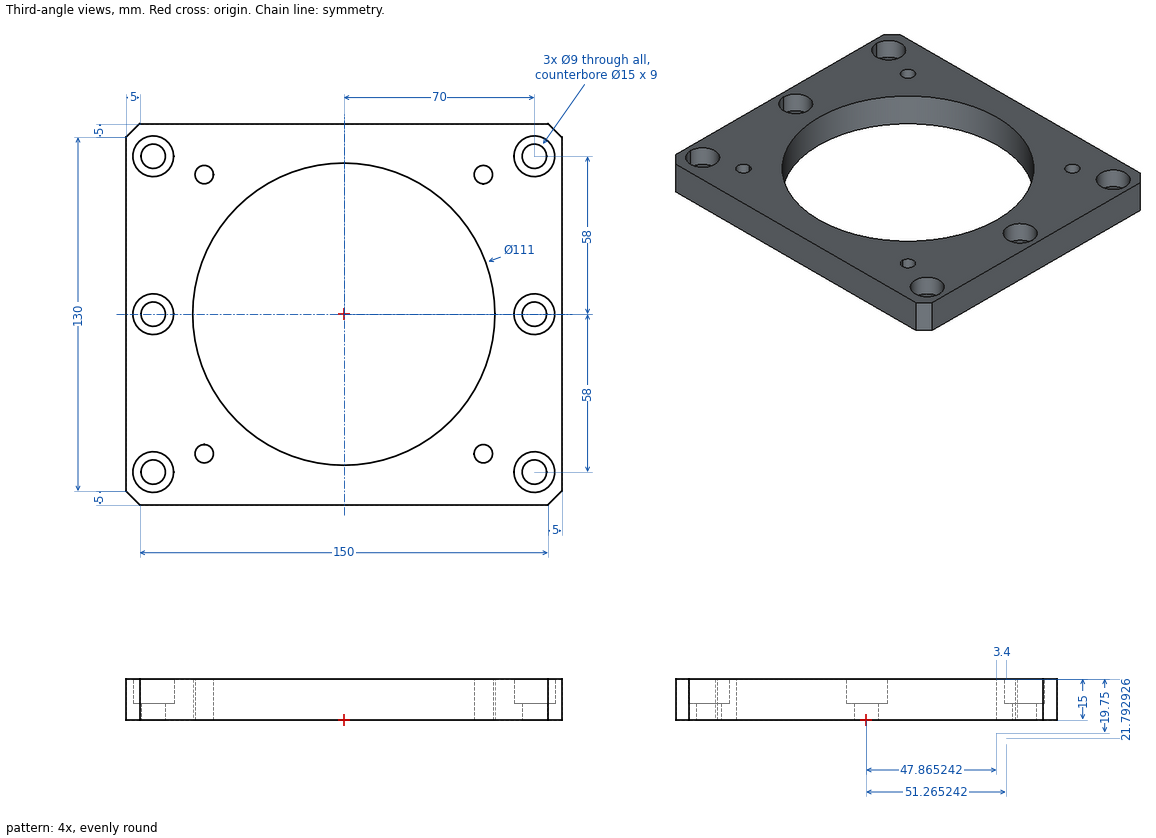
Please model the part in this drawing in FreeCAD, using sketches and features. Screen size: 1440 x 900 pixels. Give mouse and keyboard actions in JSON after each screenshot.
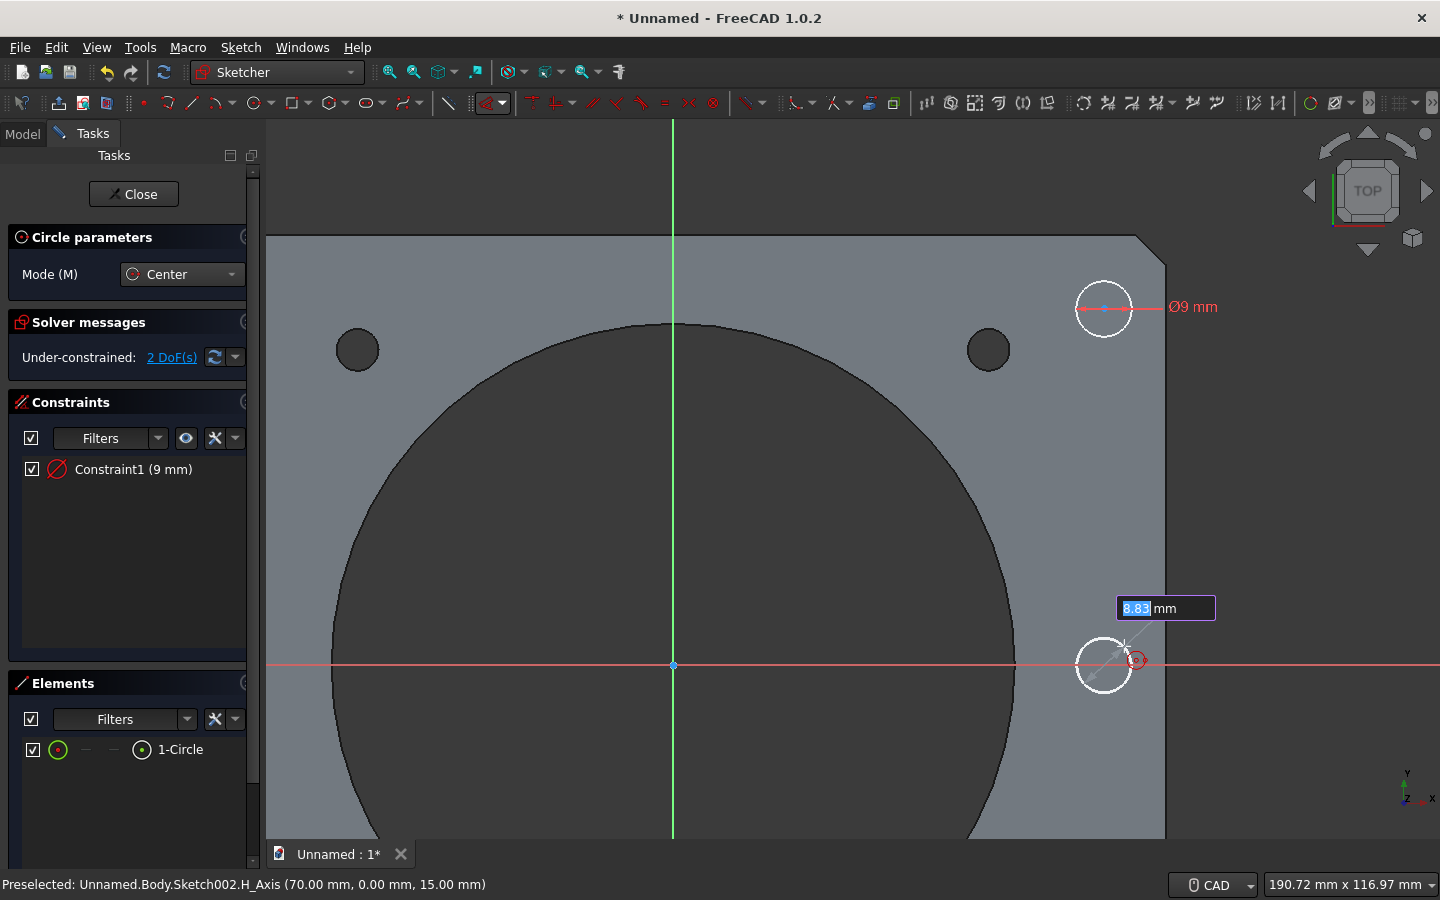
{"action": "type", "text": "9"}
{"action": "key", "text": "Return"}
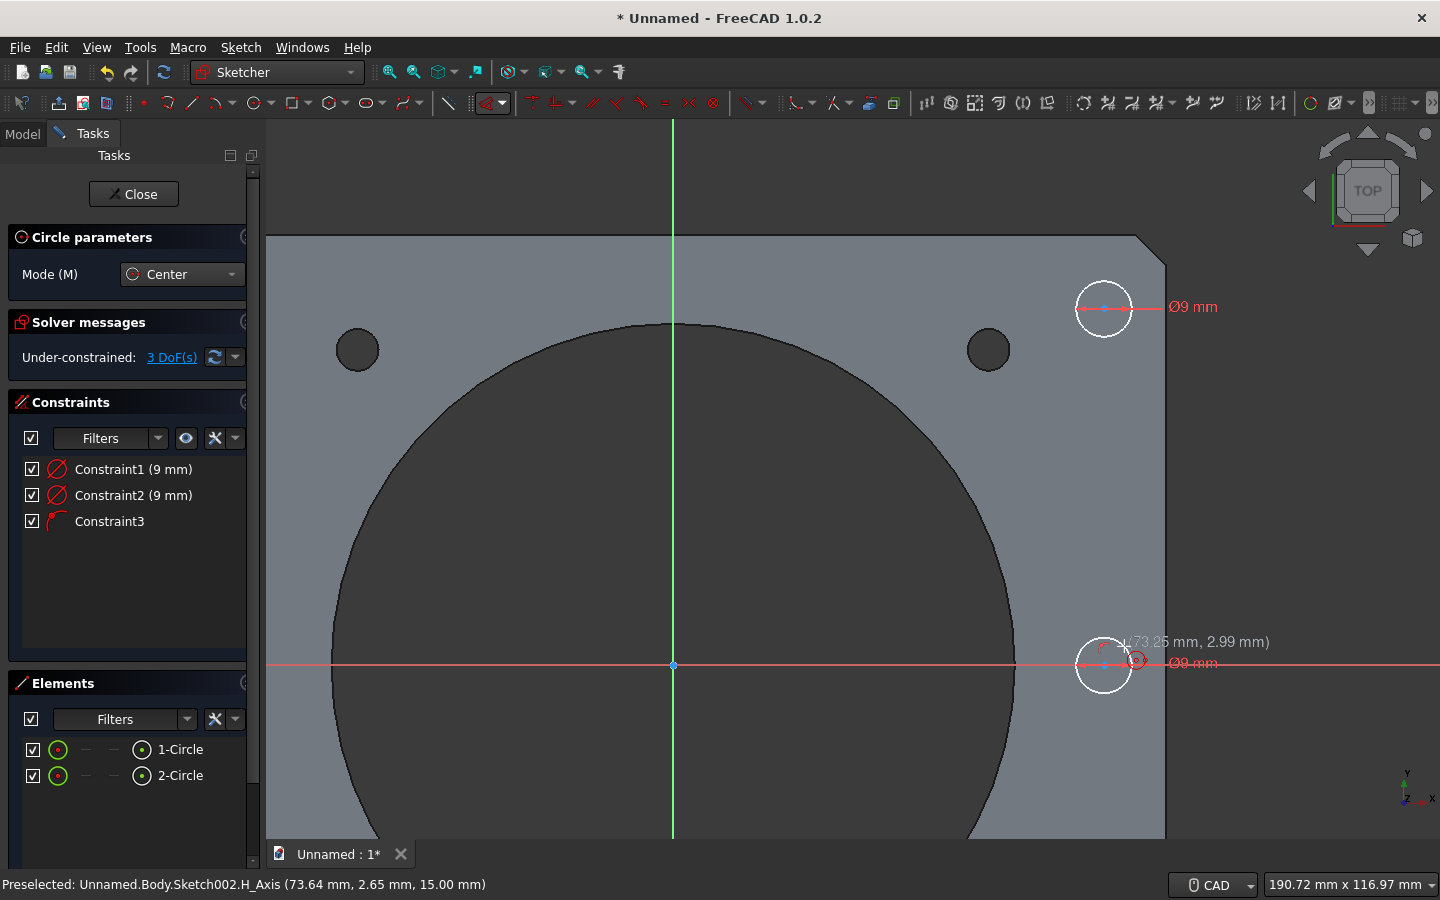
{"action": "scroll", "coordinate": [545, 147], "scroll_direction": "down", "scroll_amount": 2}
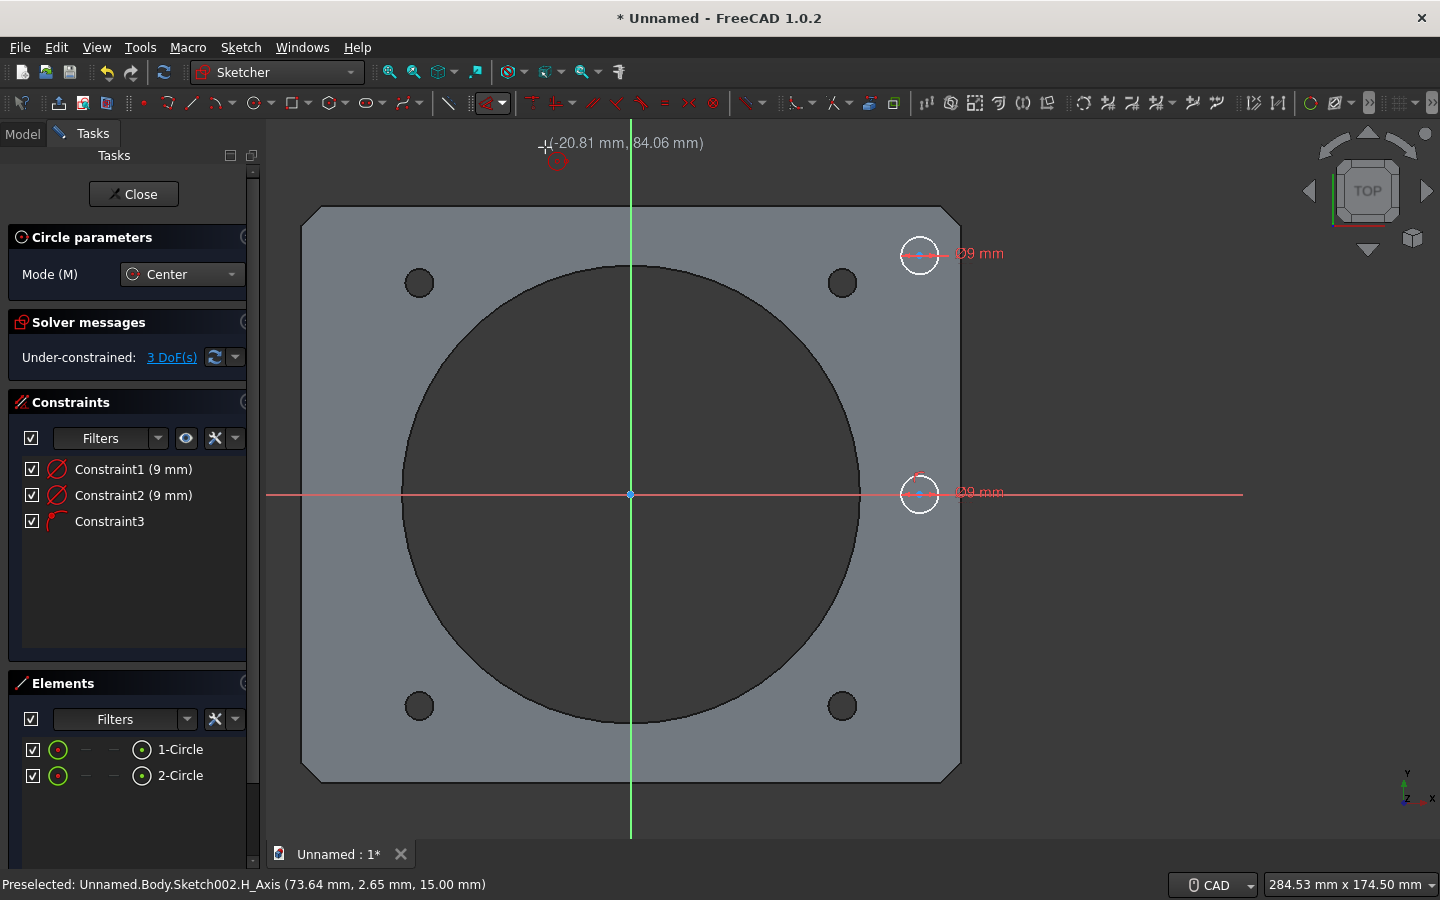
{"action": "scroll", "coordinate": [920, 734], "scroll_direction": "up", "scroll_amount": 2}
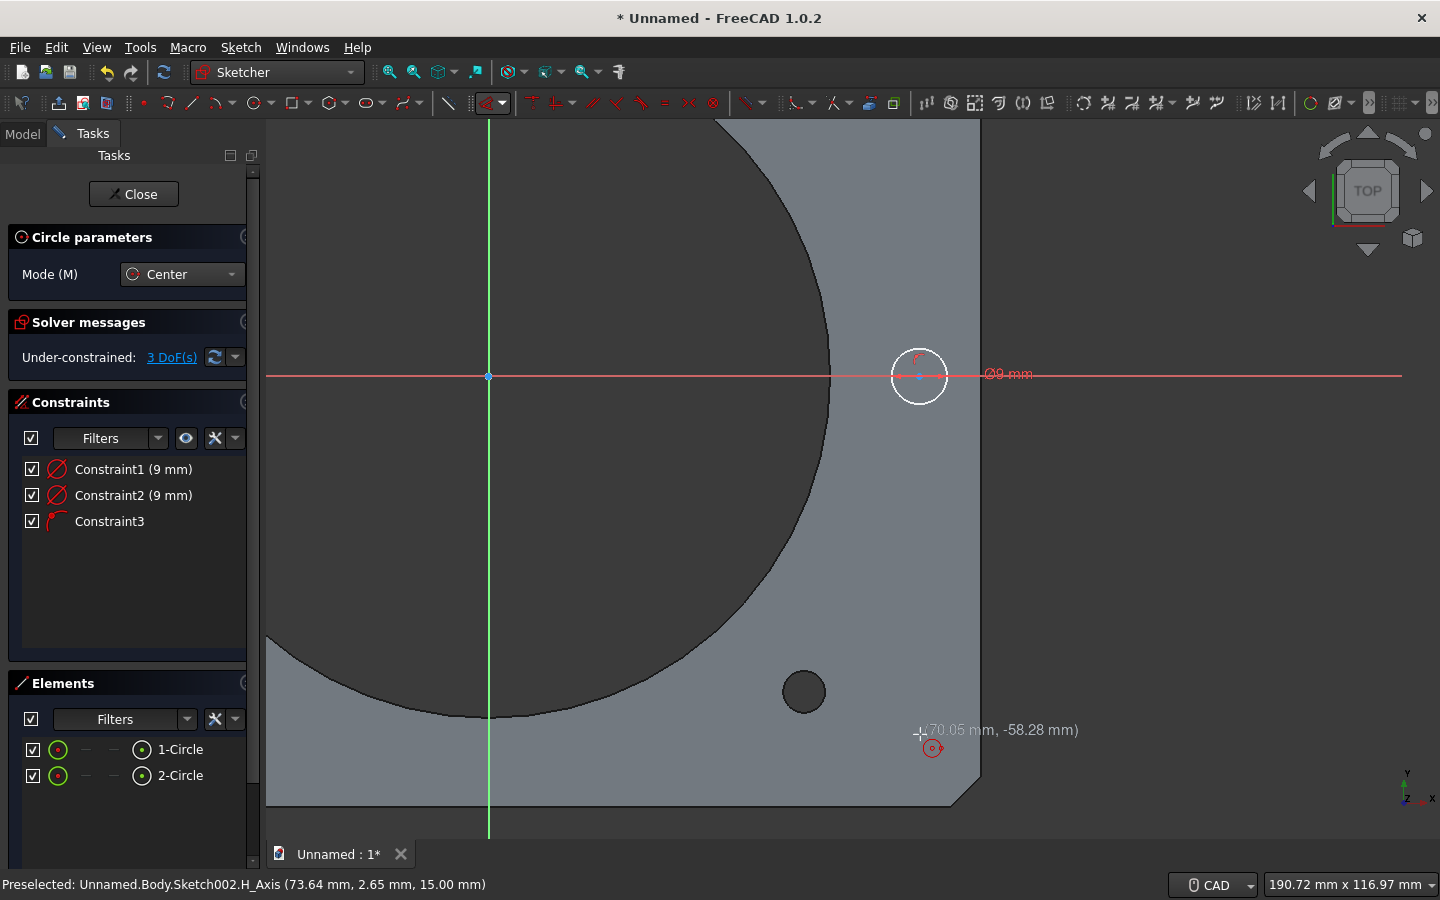
{"action": "left_click", "coordinate": [919, 733]}
{"action": "mouse_move", "coordinate": [939, 714]}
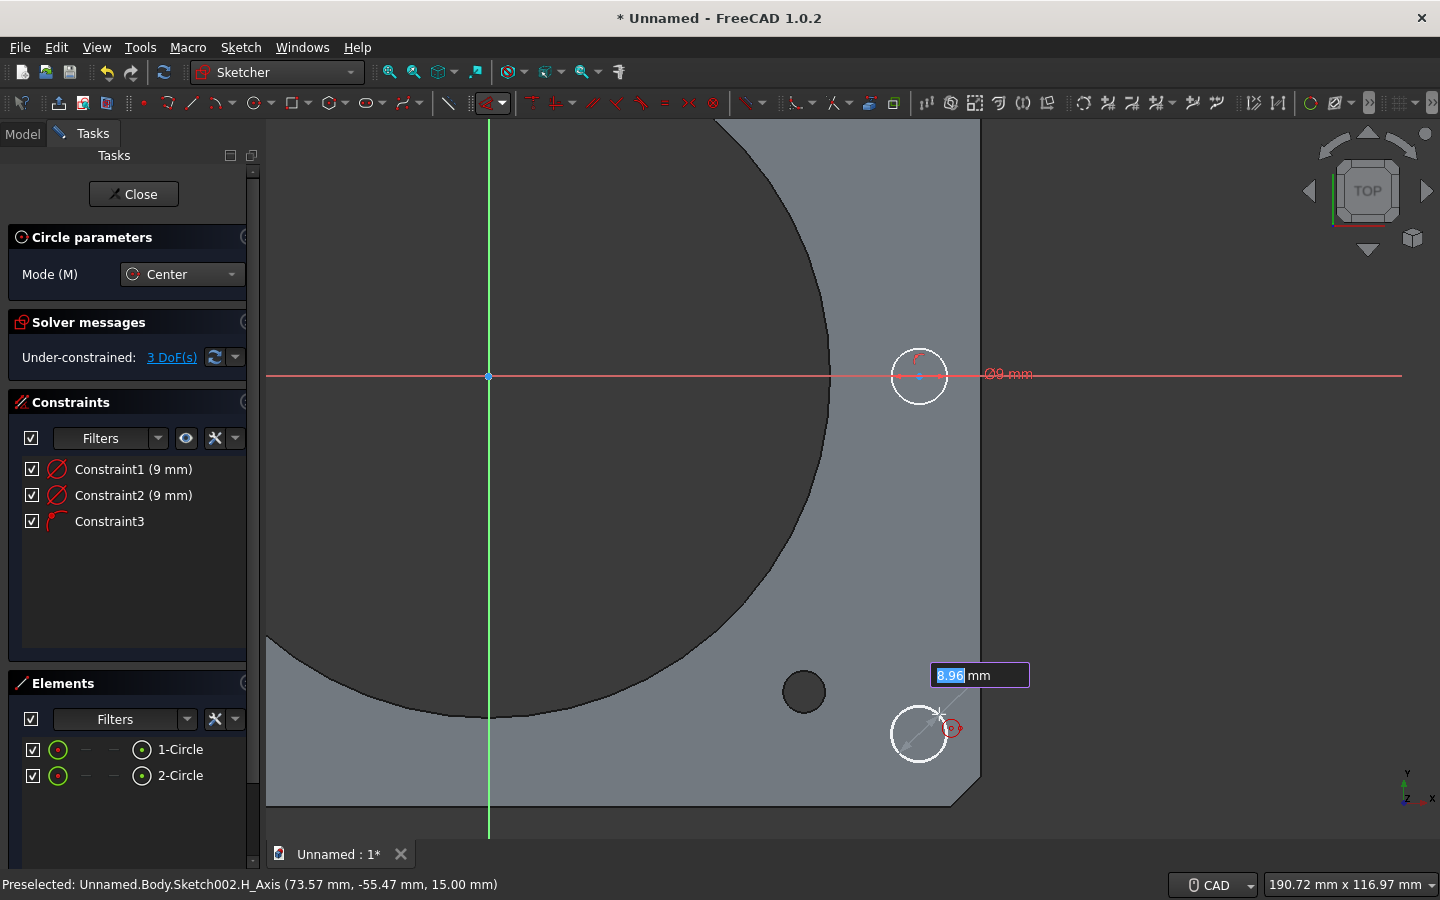
{"action": "type", "text": "9"}
{"action": "key", "text": "Return"}
{"action": "key", "text": "Escape"}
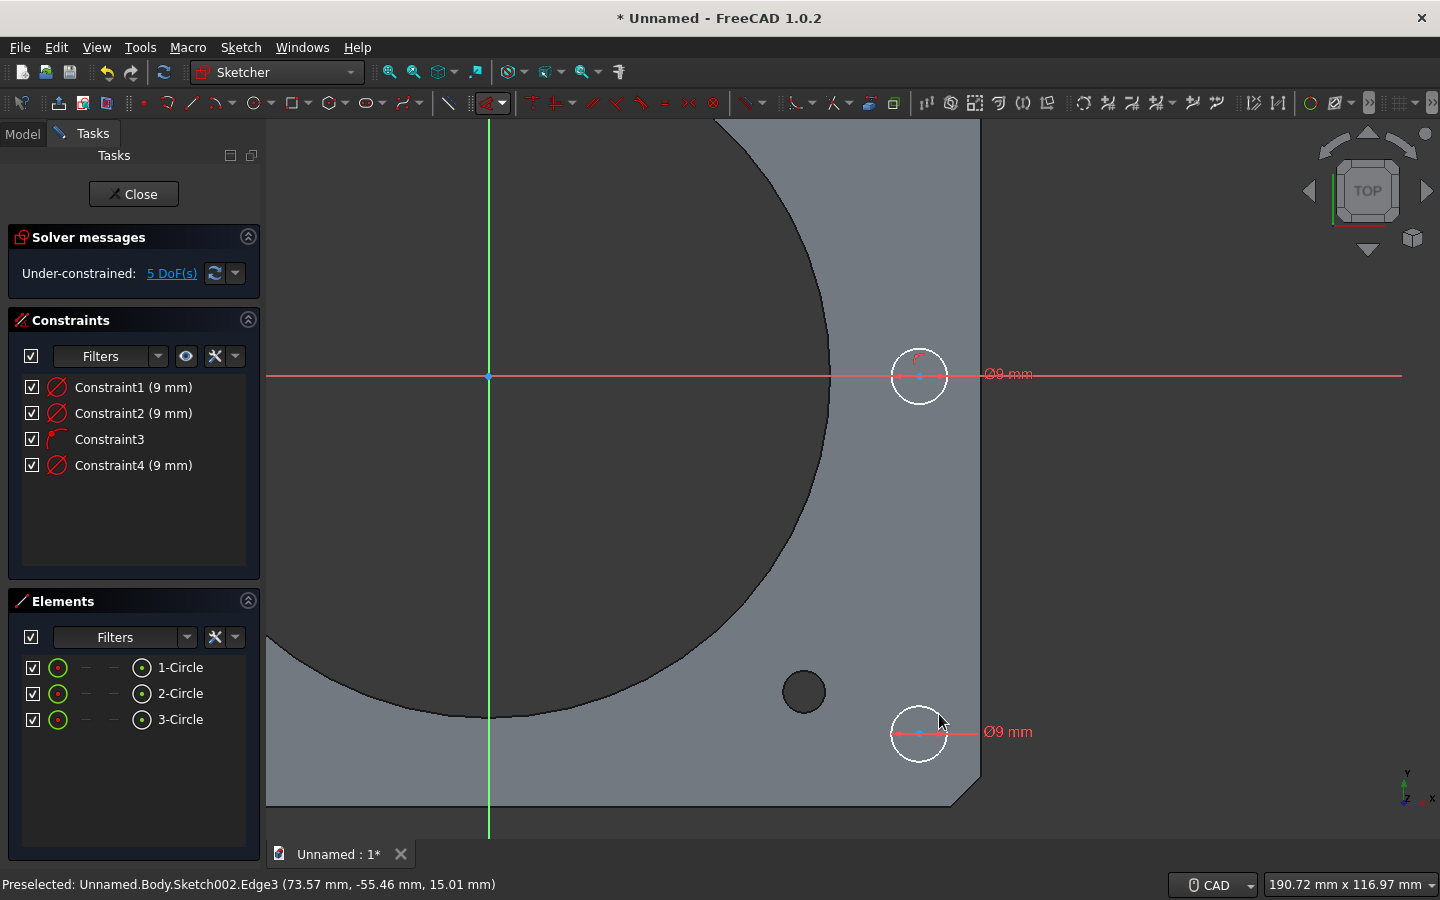
{"action": "scroll", "coordinate": [920, 688], "scroll_direction": "down", "scroll_amount": 2}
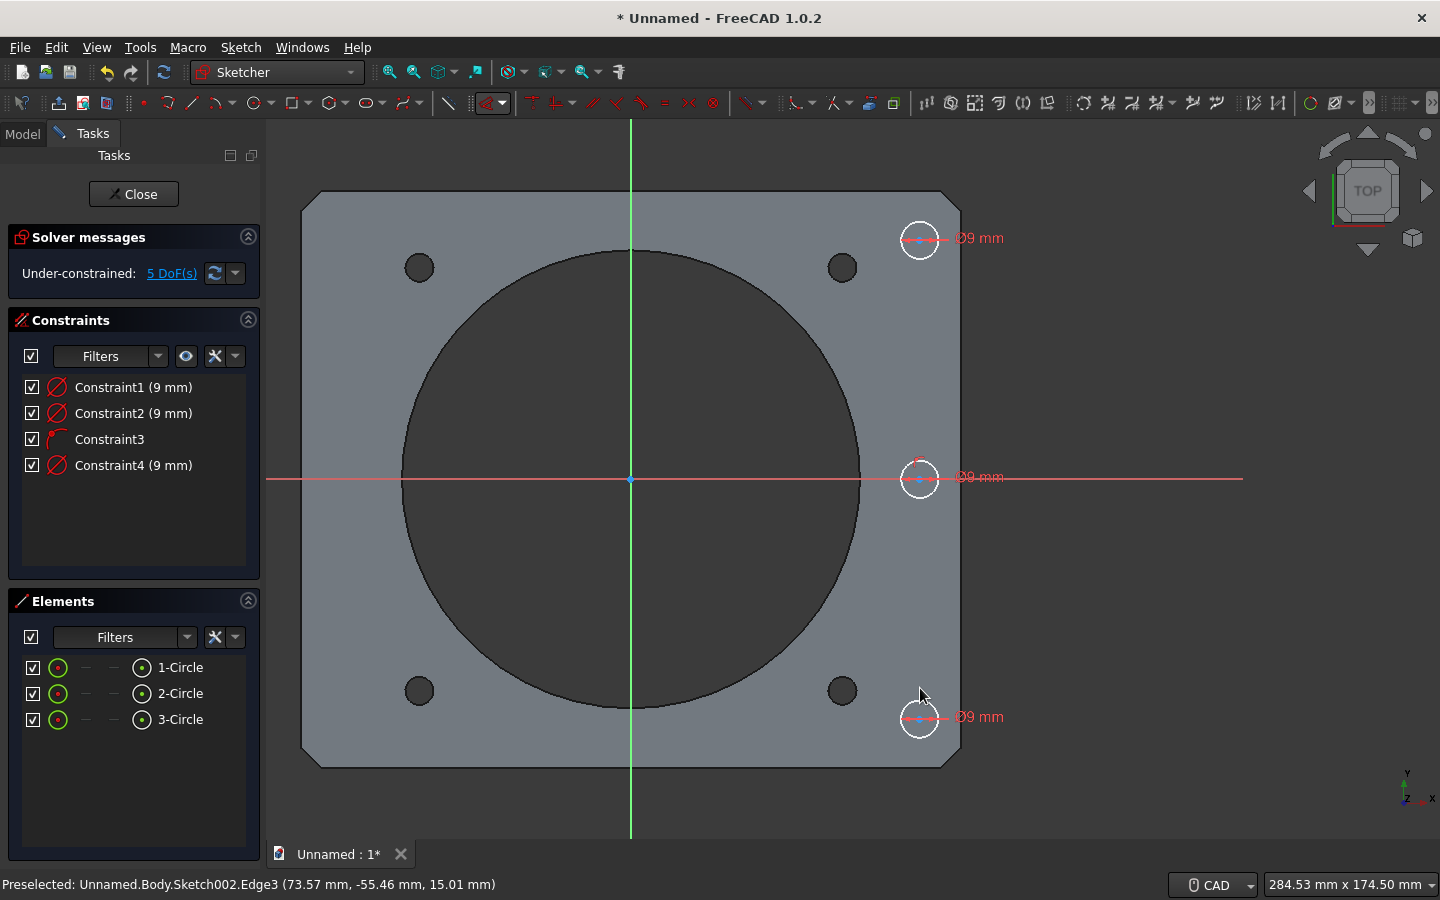
{"action": "left_click", "coordinate": [920, 240]}